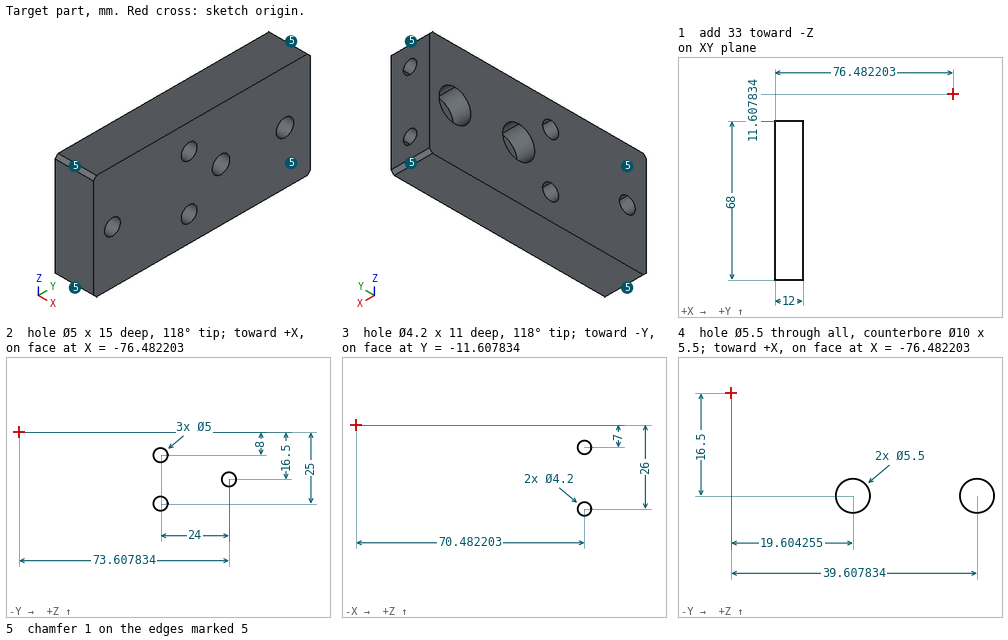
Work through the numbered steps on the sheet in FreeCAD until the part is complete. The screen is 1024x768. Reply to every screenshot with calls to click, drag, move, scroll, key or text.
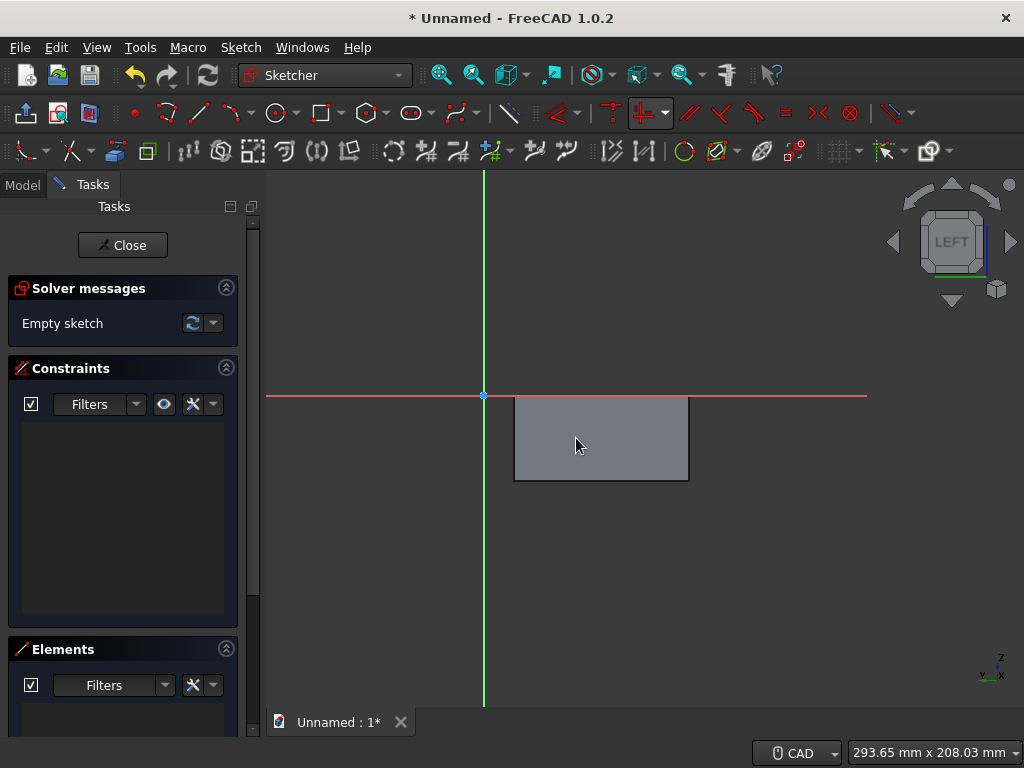
scroll(660, 438, up, 8)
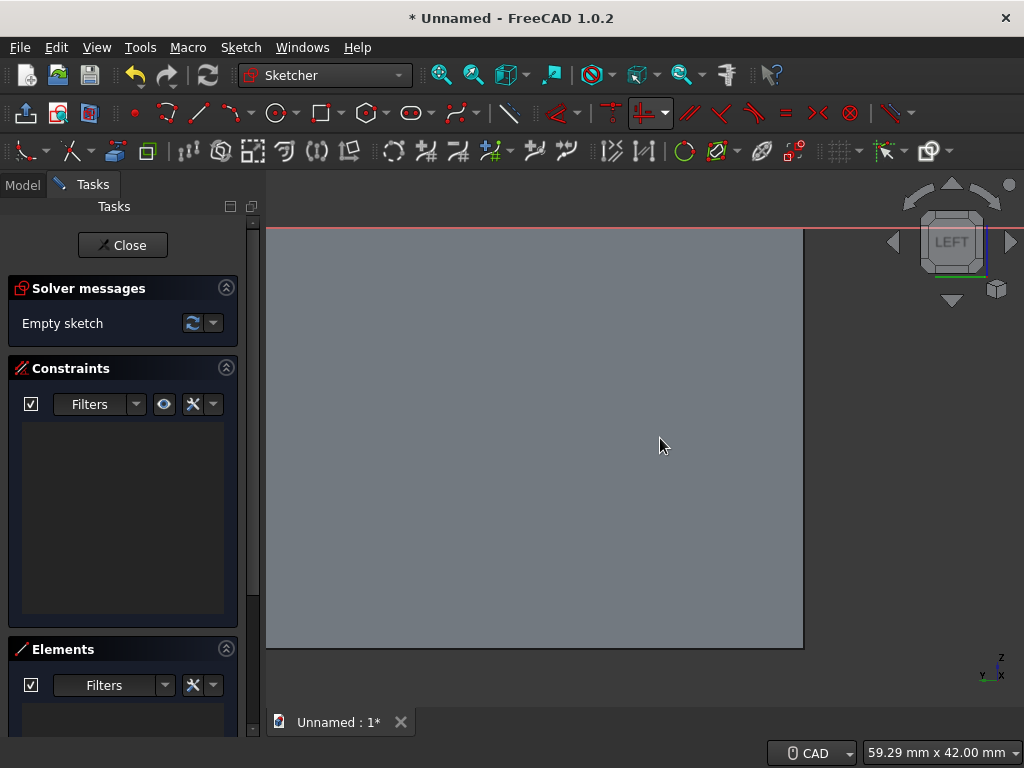
key(g)
key(c)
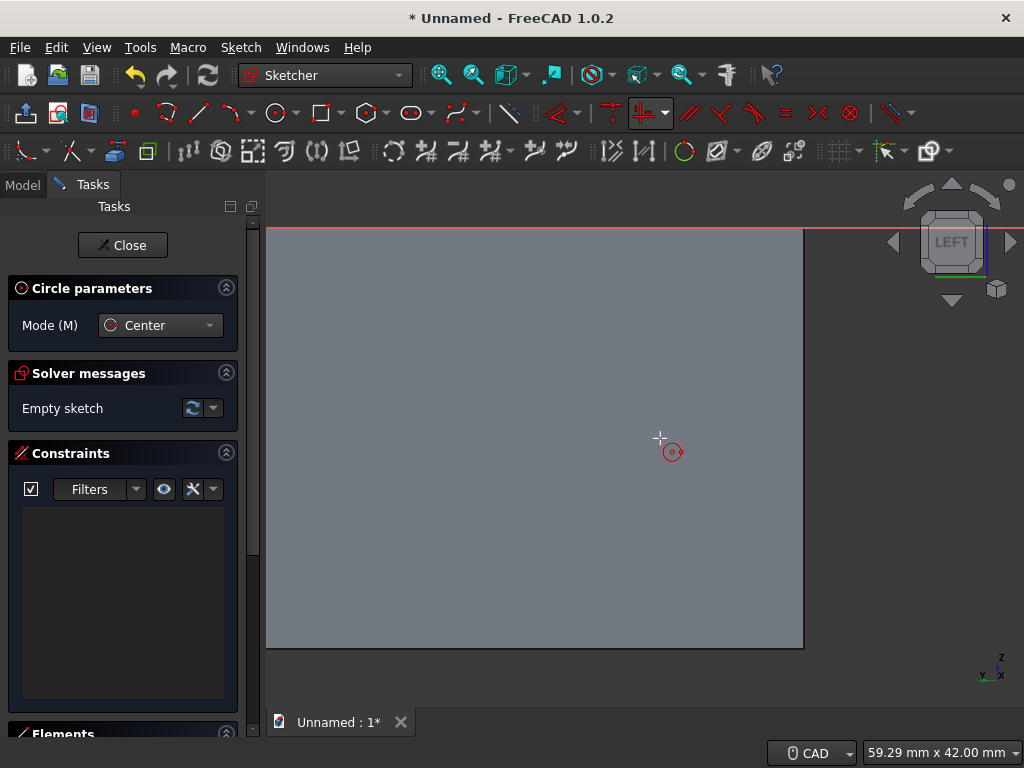
click(727, 438)
click(749, 416)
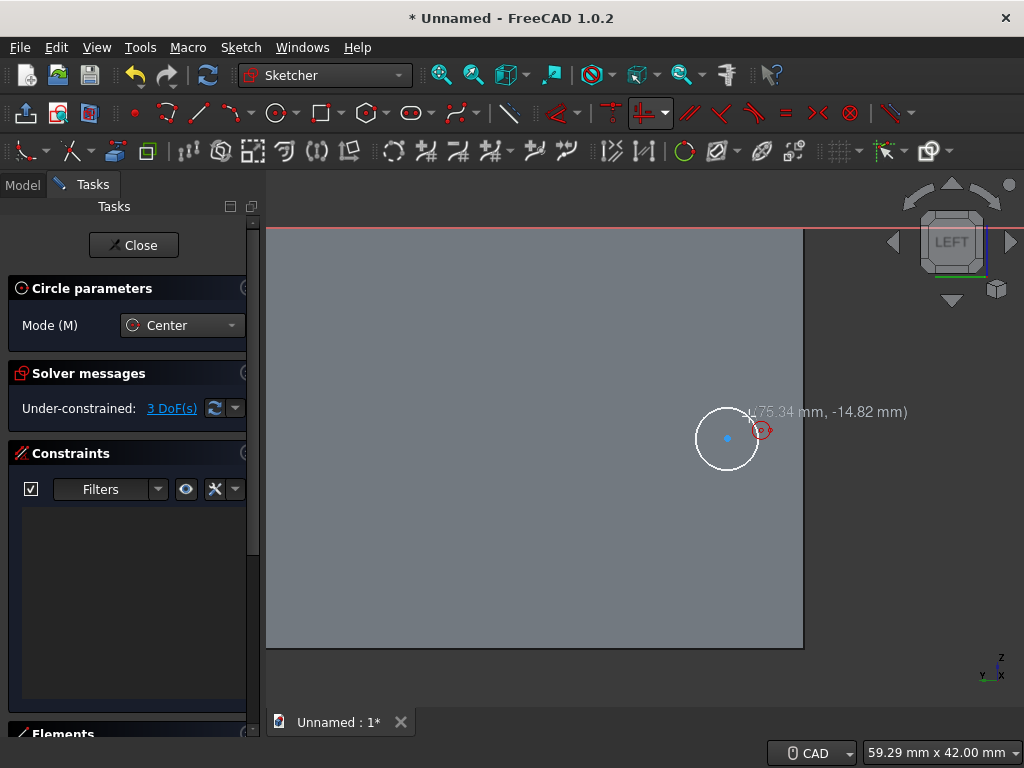
click(420, 330)
click(443, 307)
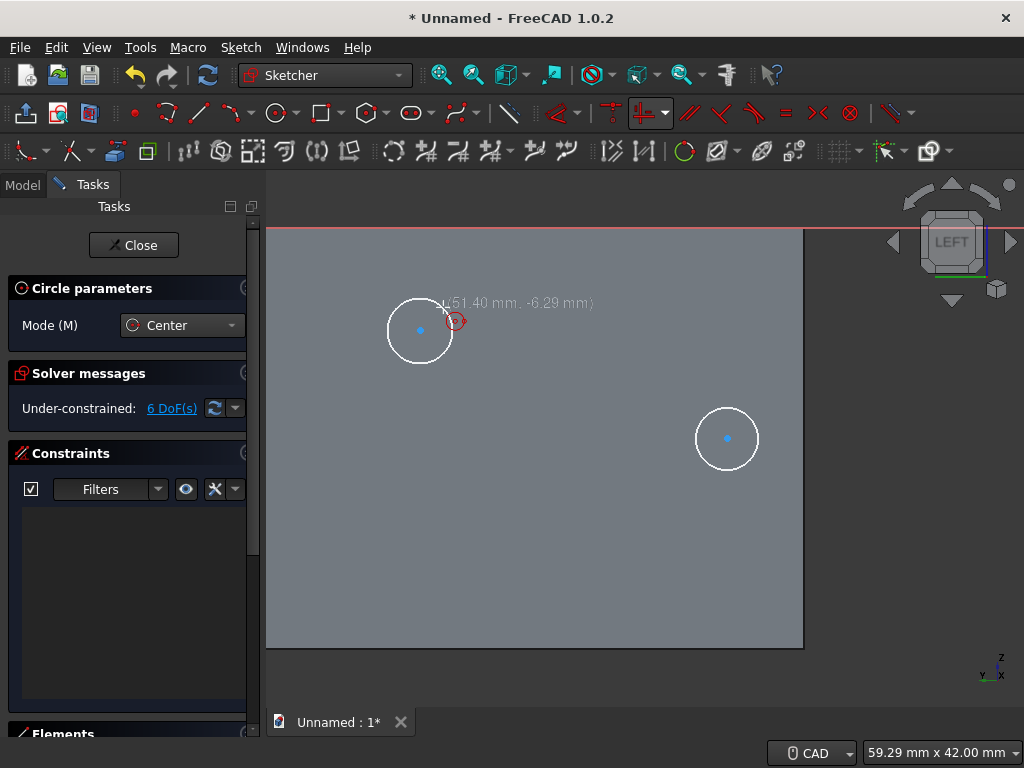
click(420, 547)
click(443, 525)
key(Escape)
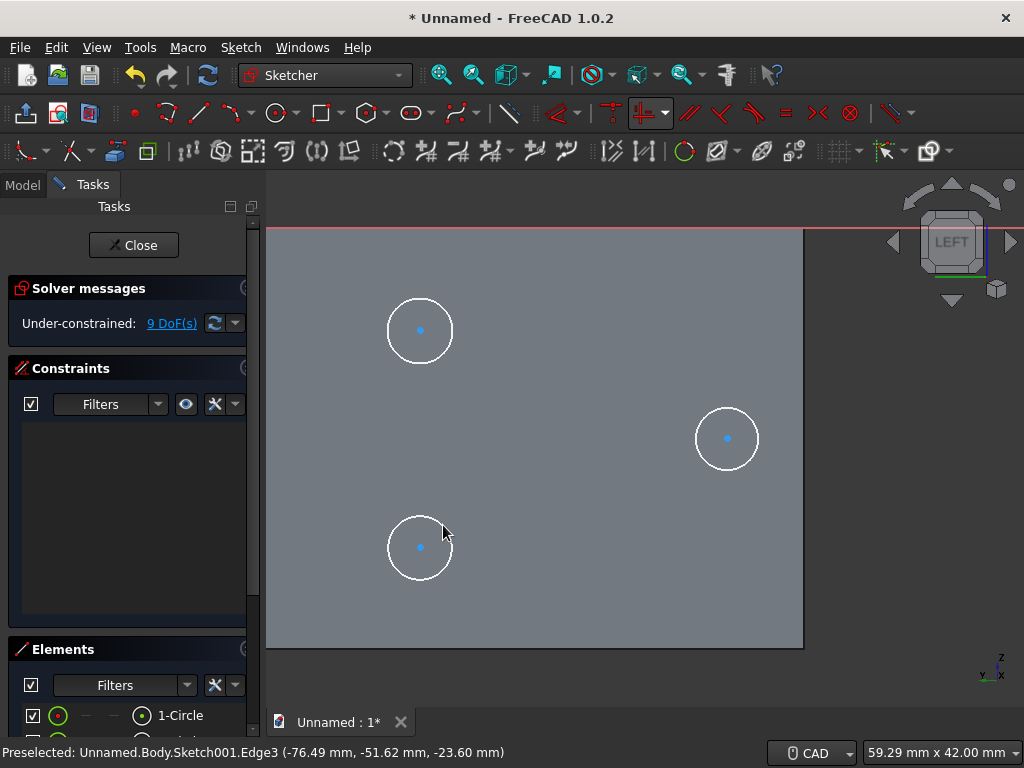
click(749, 417)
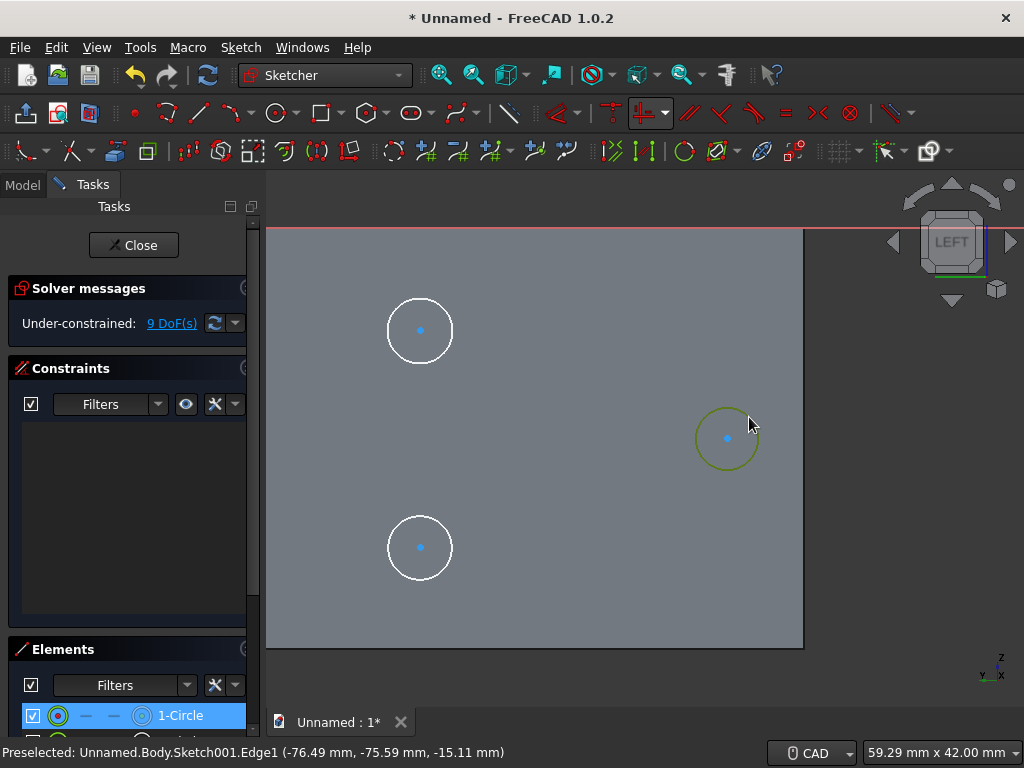
click(443, 308)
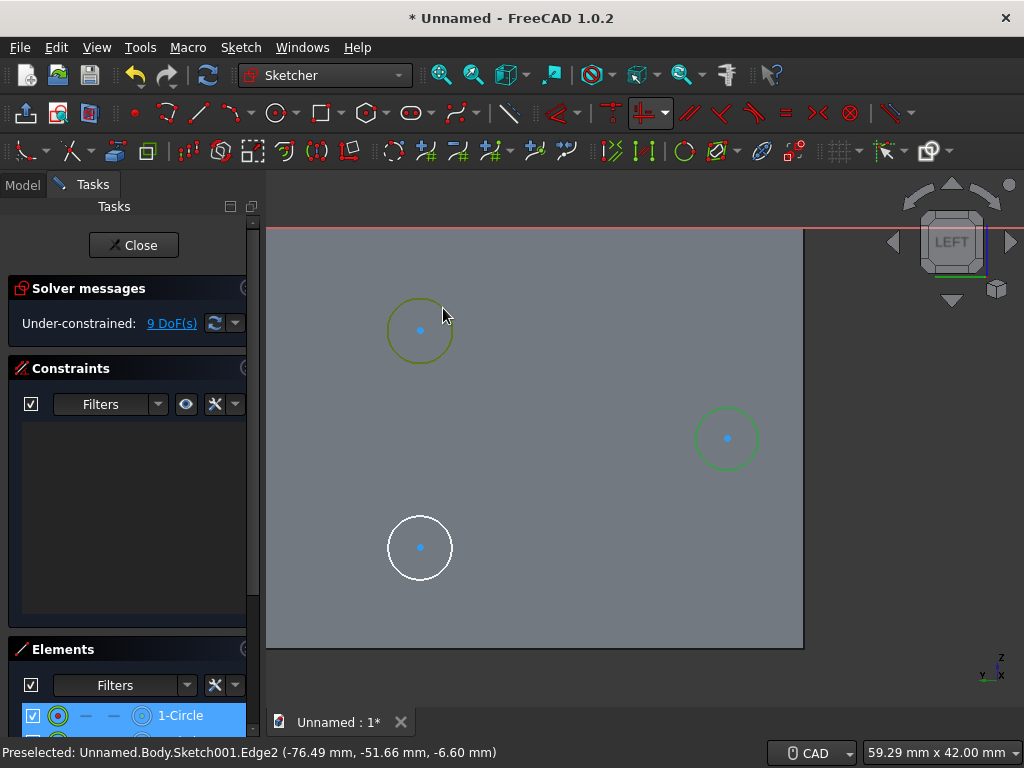
click(442, 525)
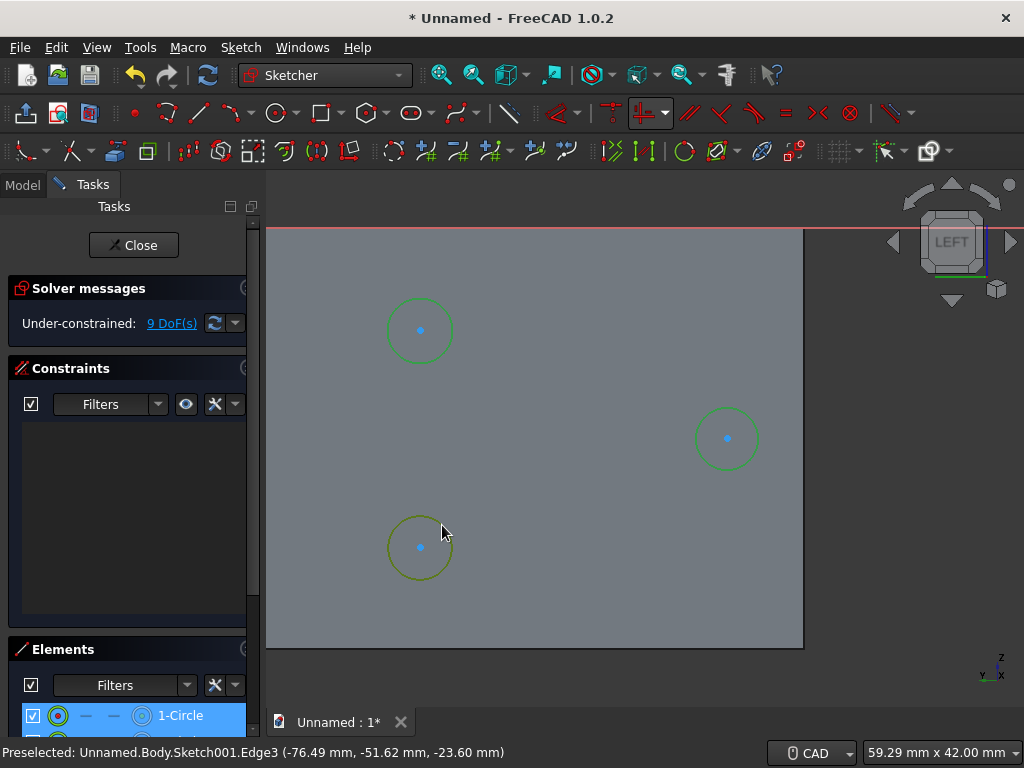
key(e)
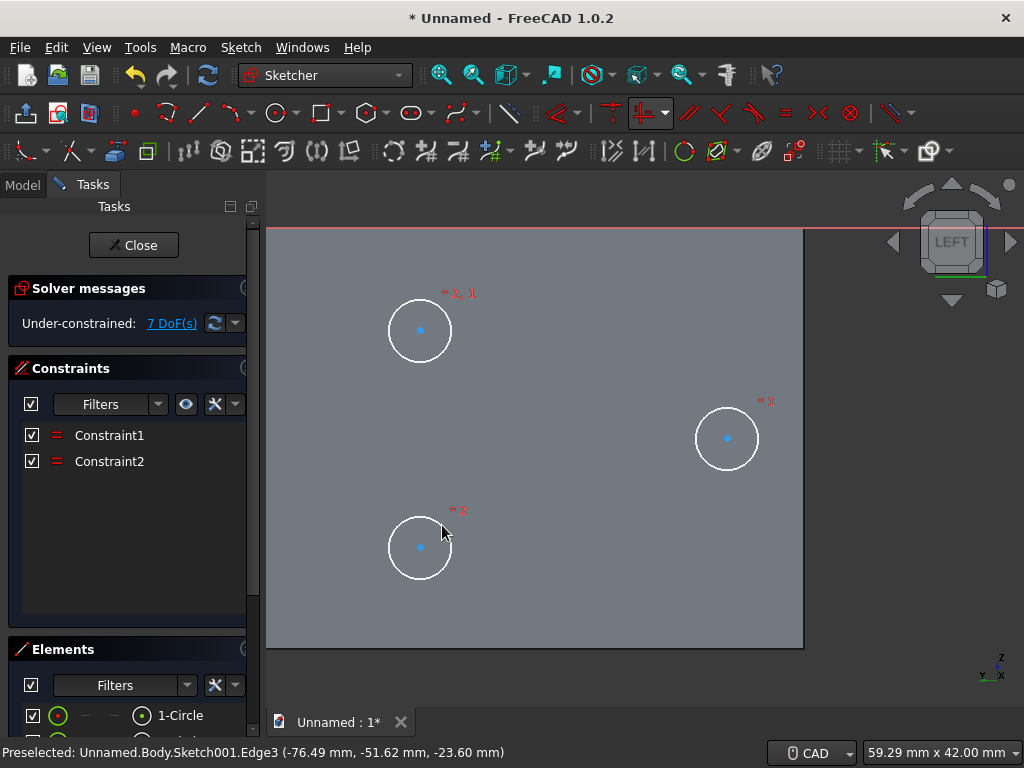
click(420, 331)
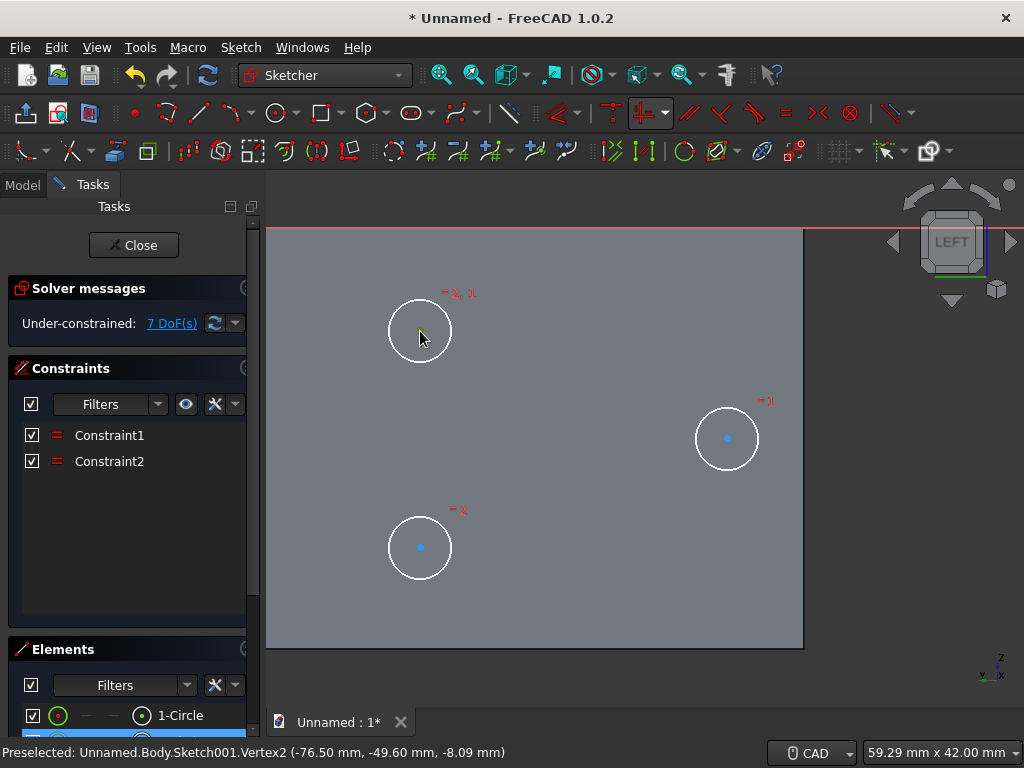
click(420, 548)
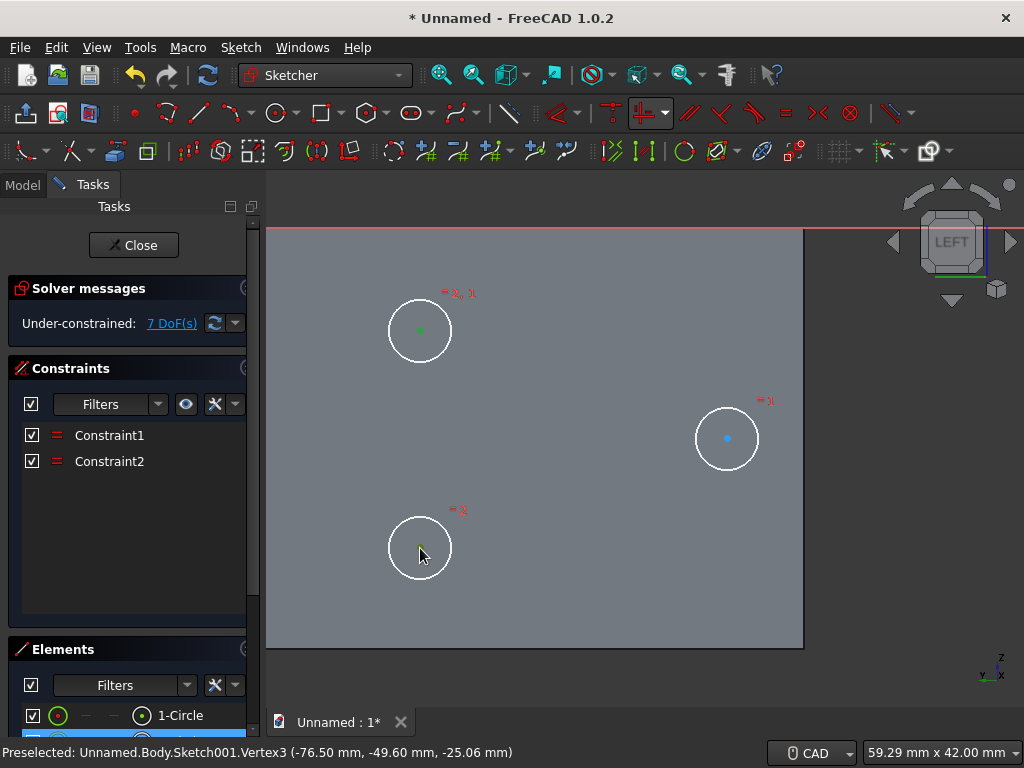
key(v)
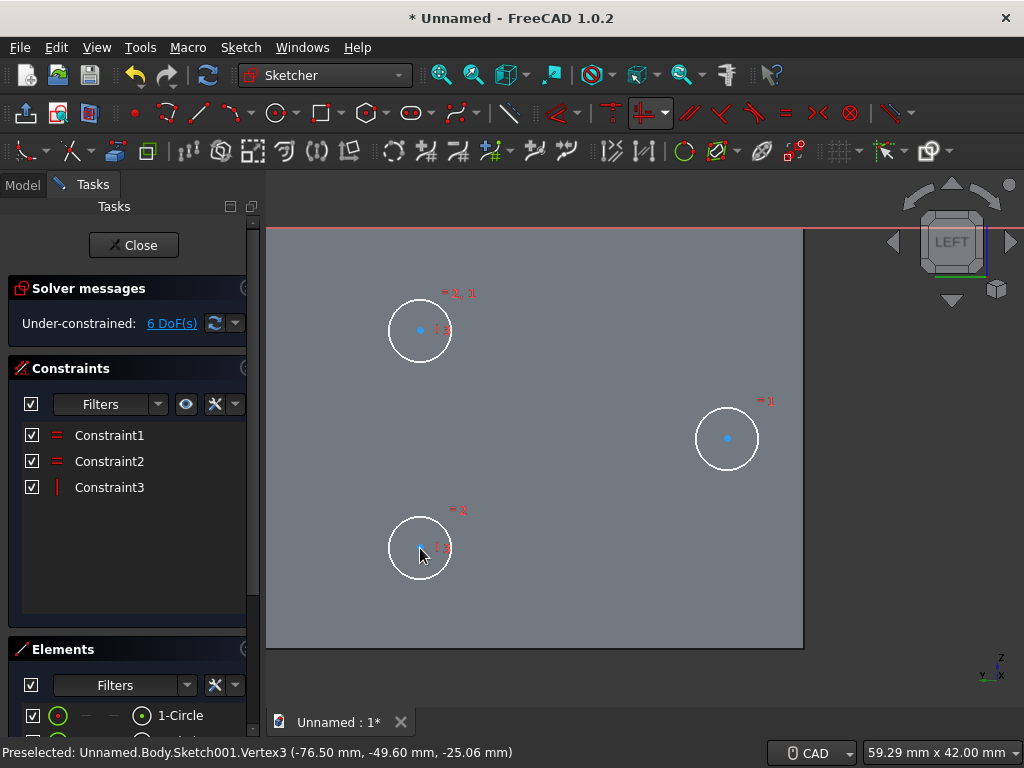
key(d)